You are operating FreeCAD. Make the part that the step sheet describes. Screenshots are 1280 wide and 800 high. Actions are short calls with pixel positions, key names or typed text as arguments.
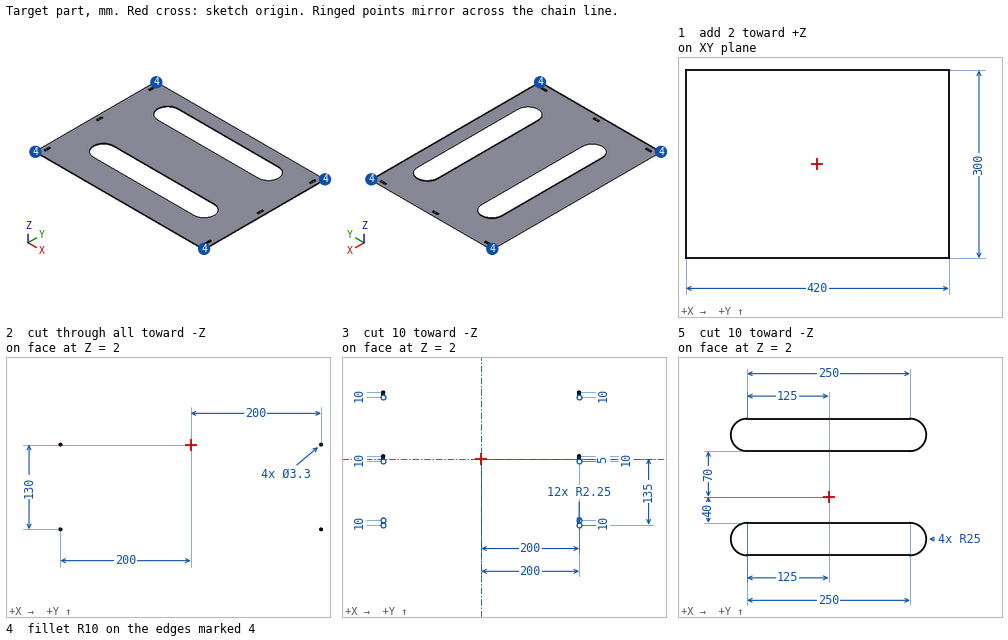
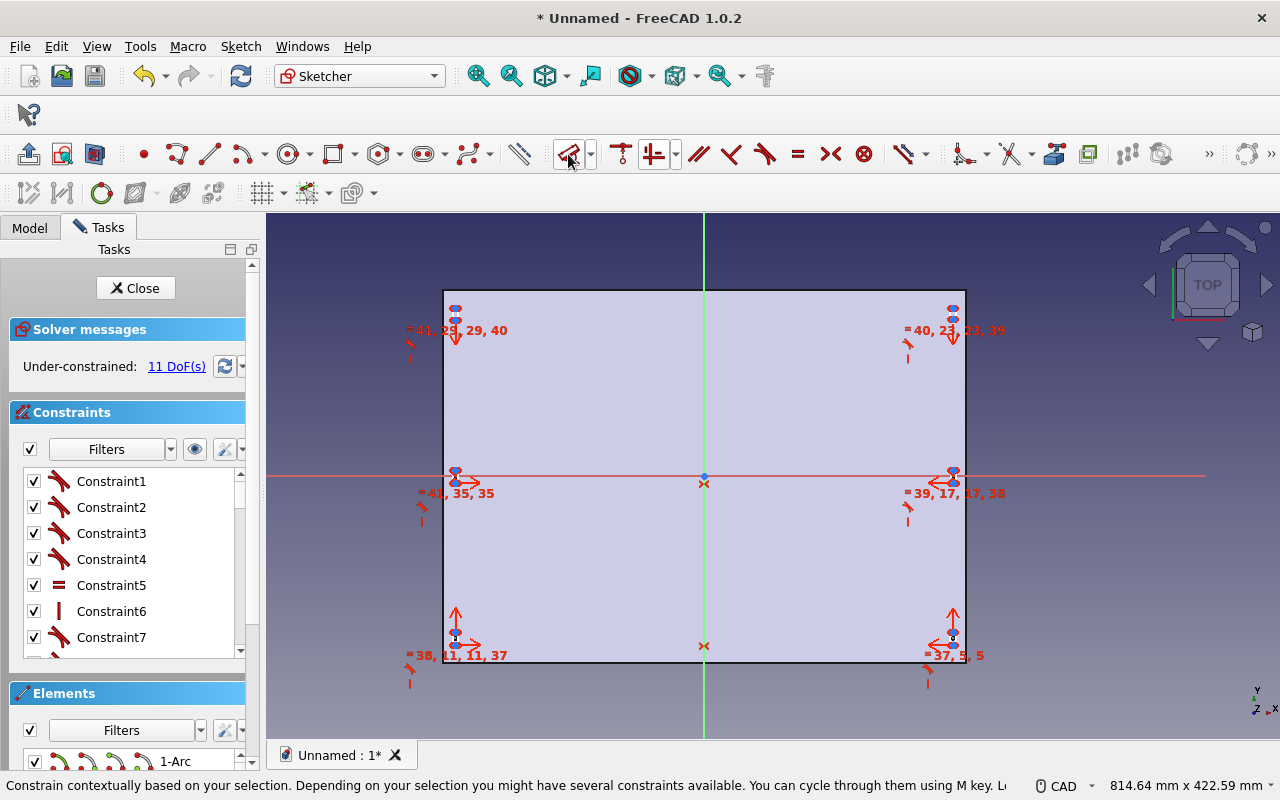
scroll(953, 648, up, 14)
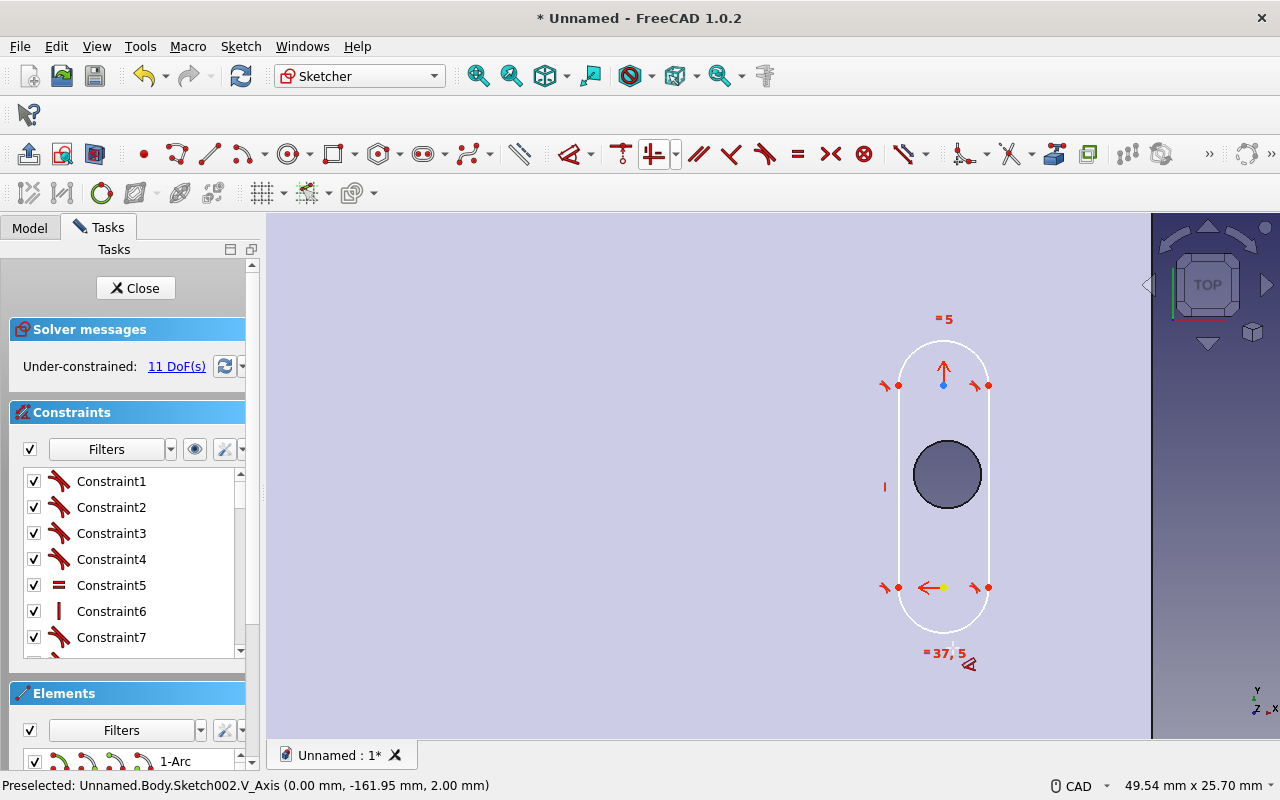
click(944, 633)
click(944, 665)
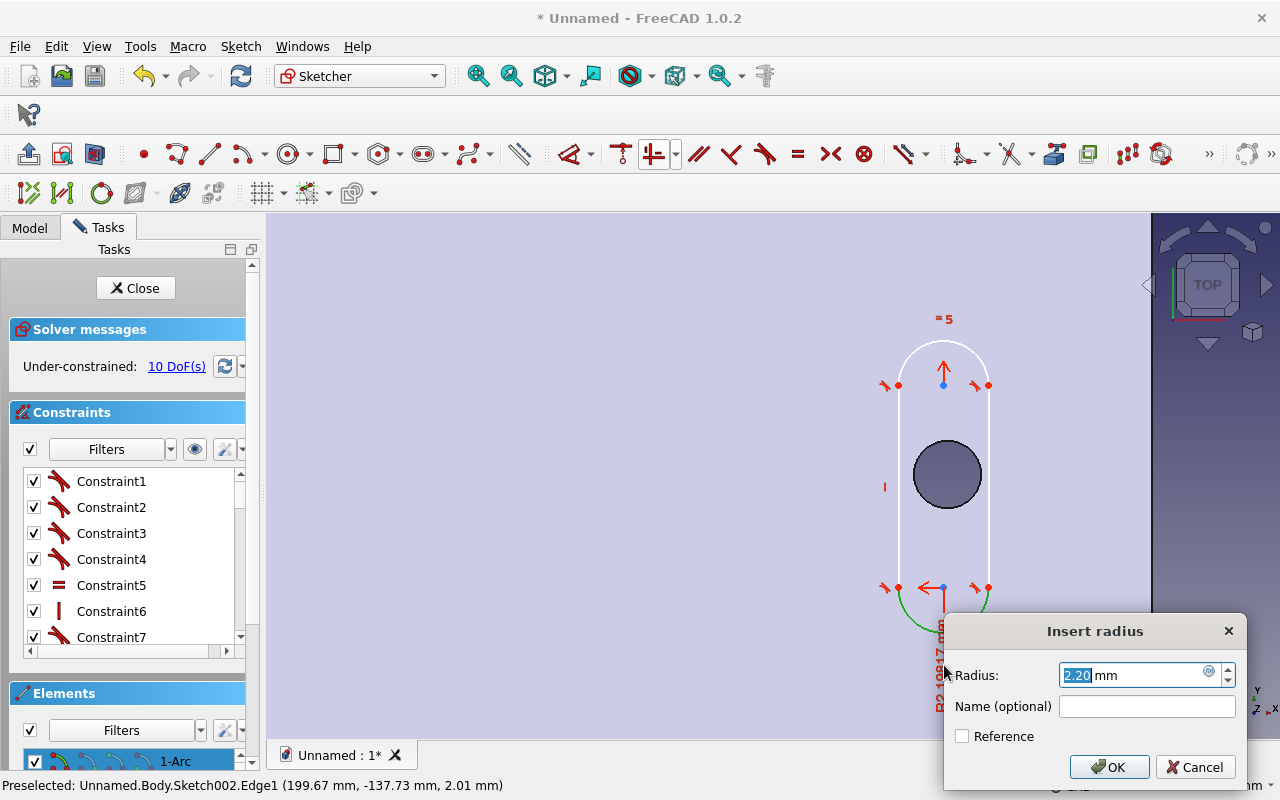
text(2.25)
key(Return)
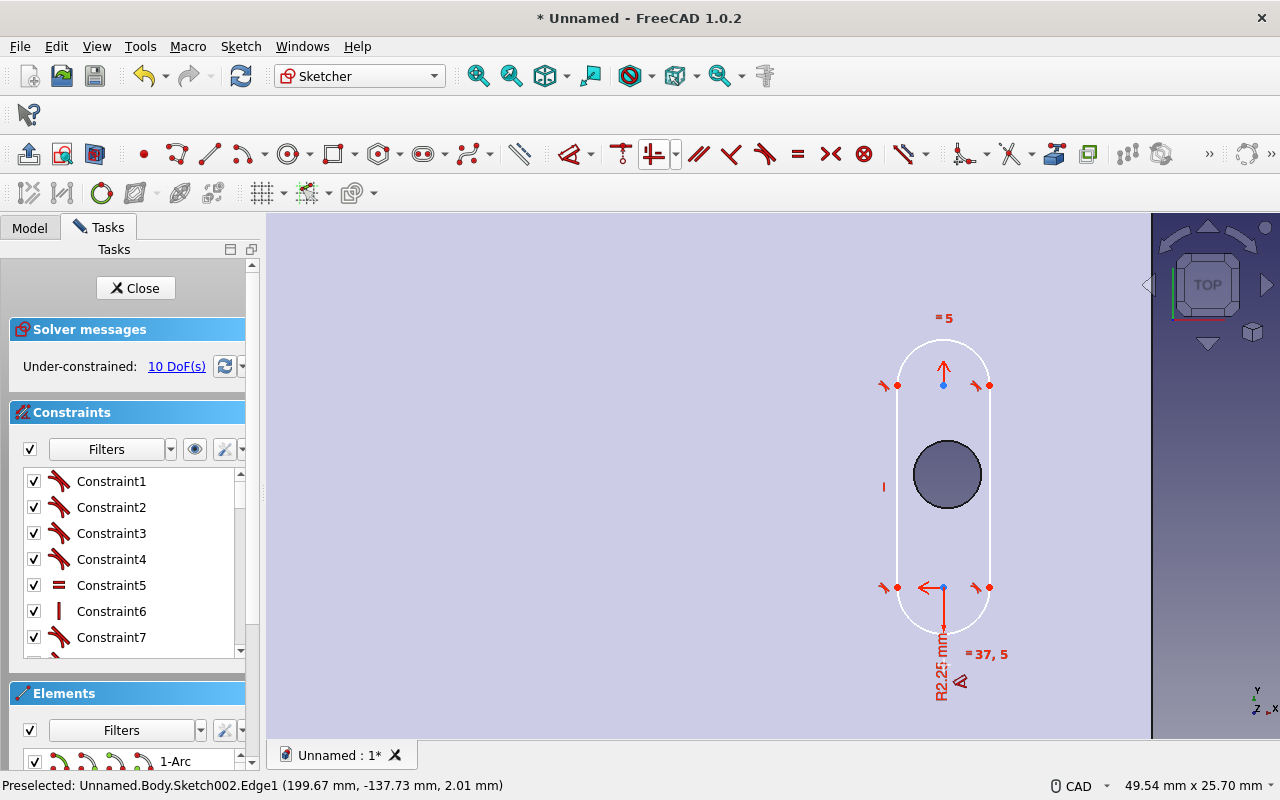
scroll(954, 648, down, 14)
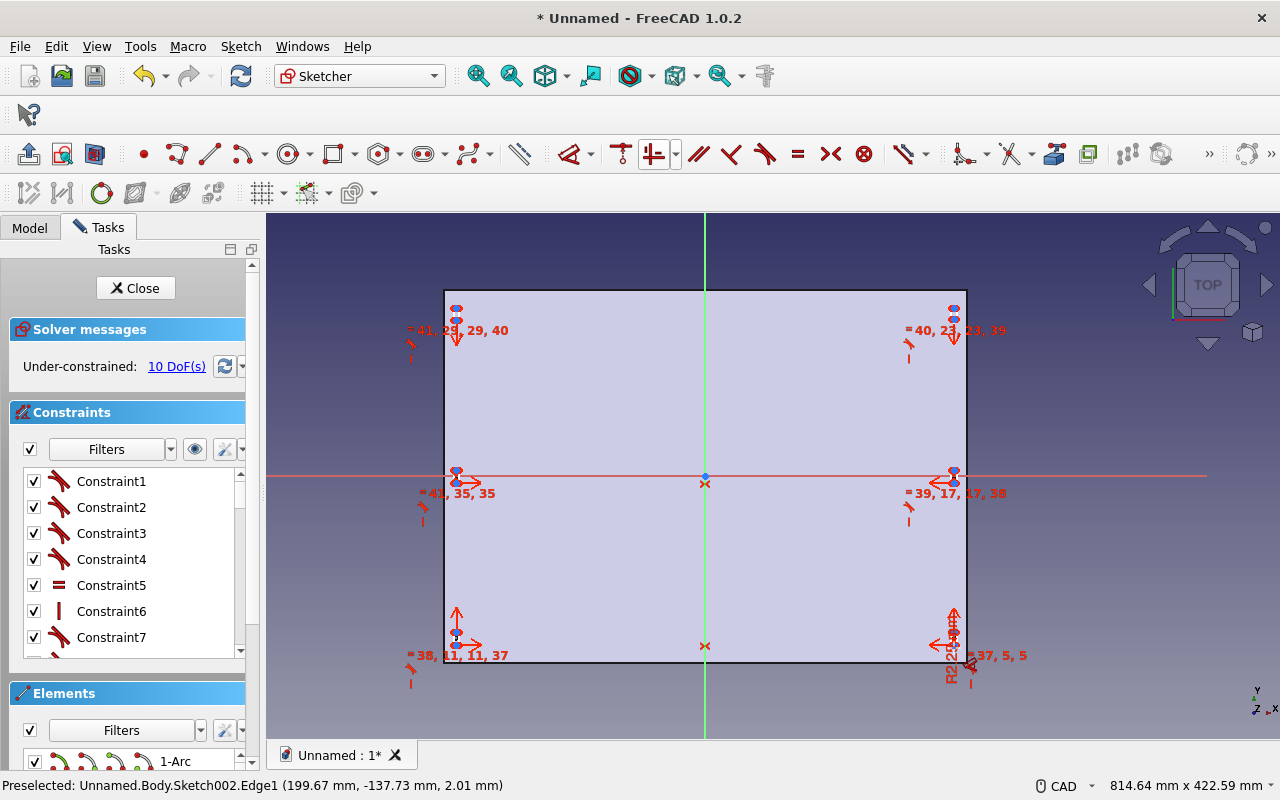
scroll(951, 641, up, 7)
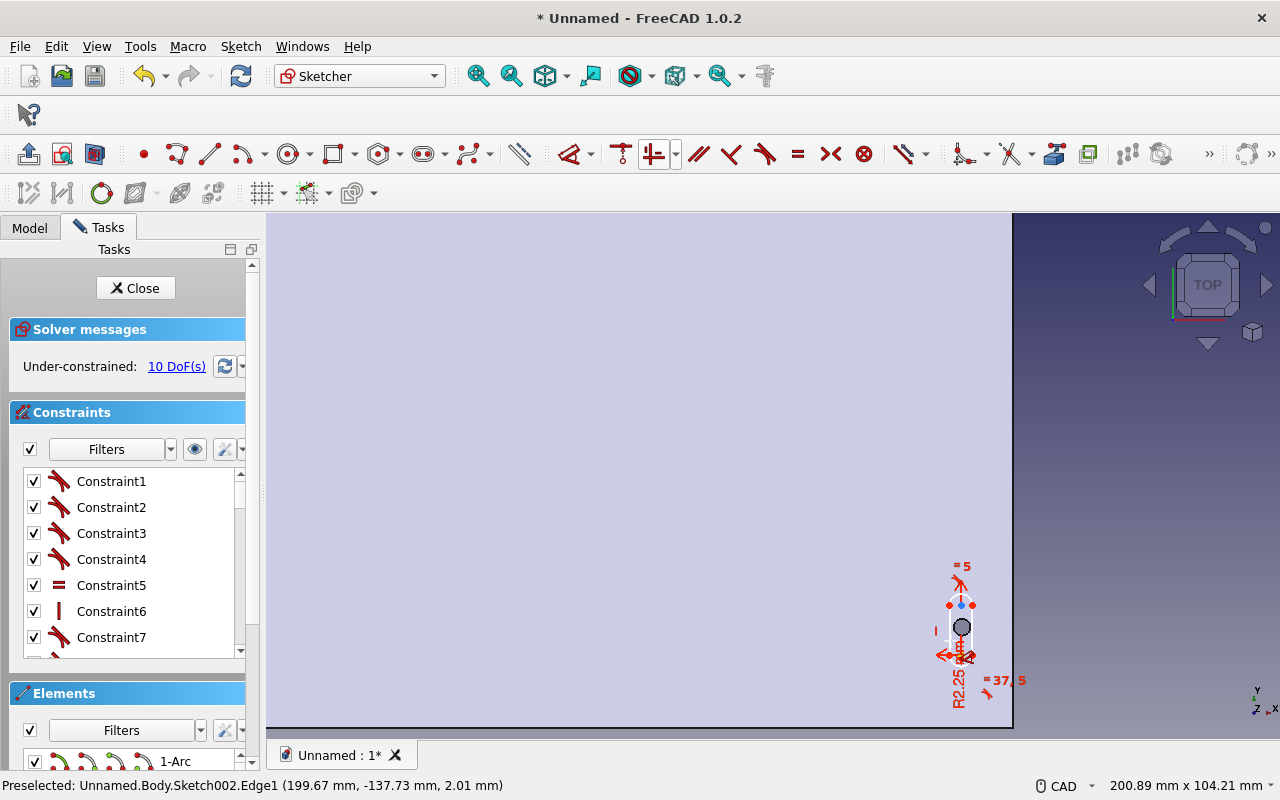
click(950, 640)
click(916, 630)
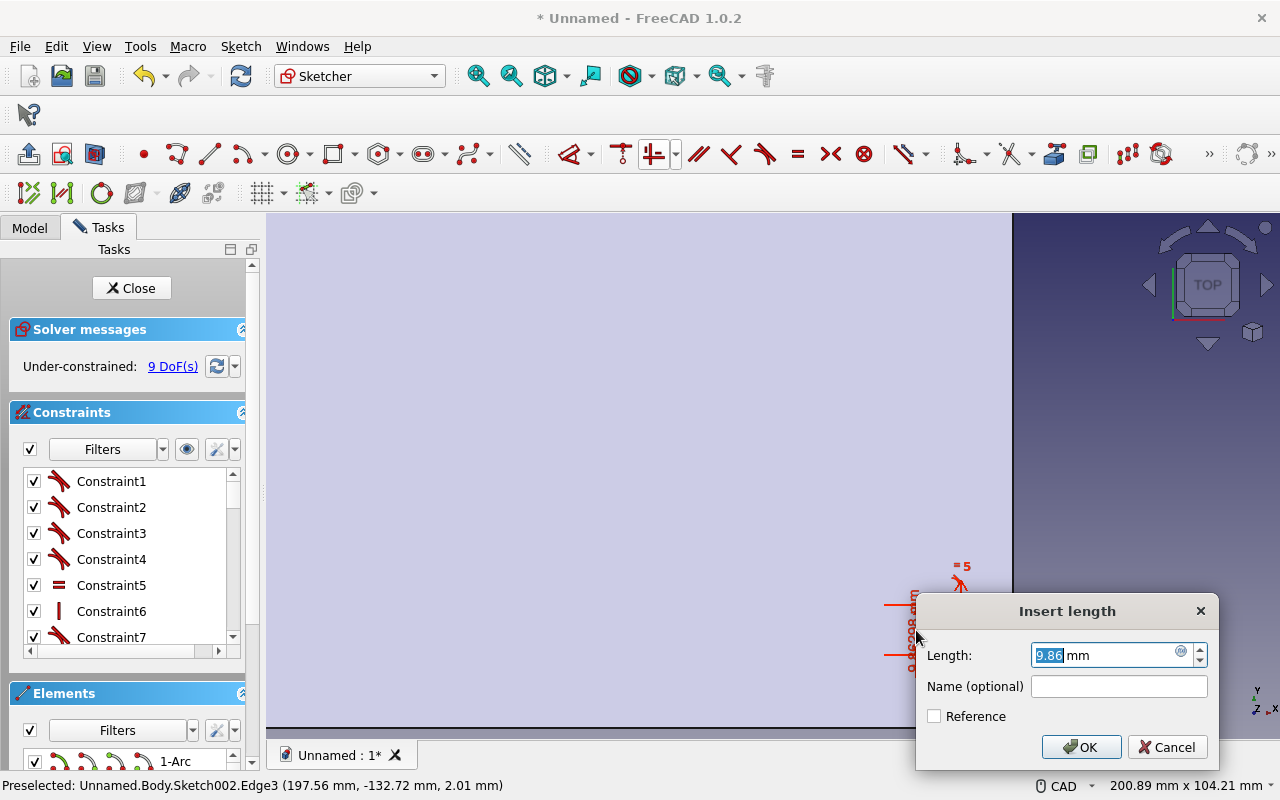
text(10)
key(Return)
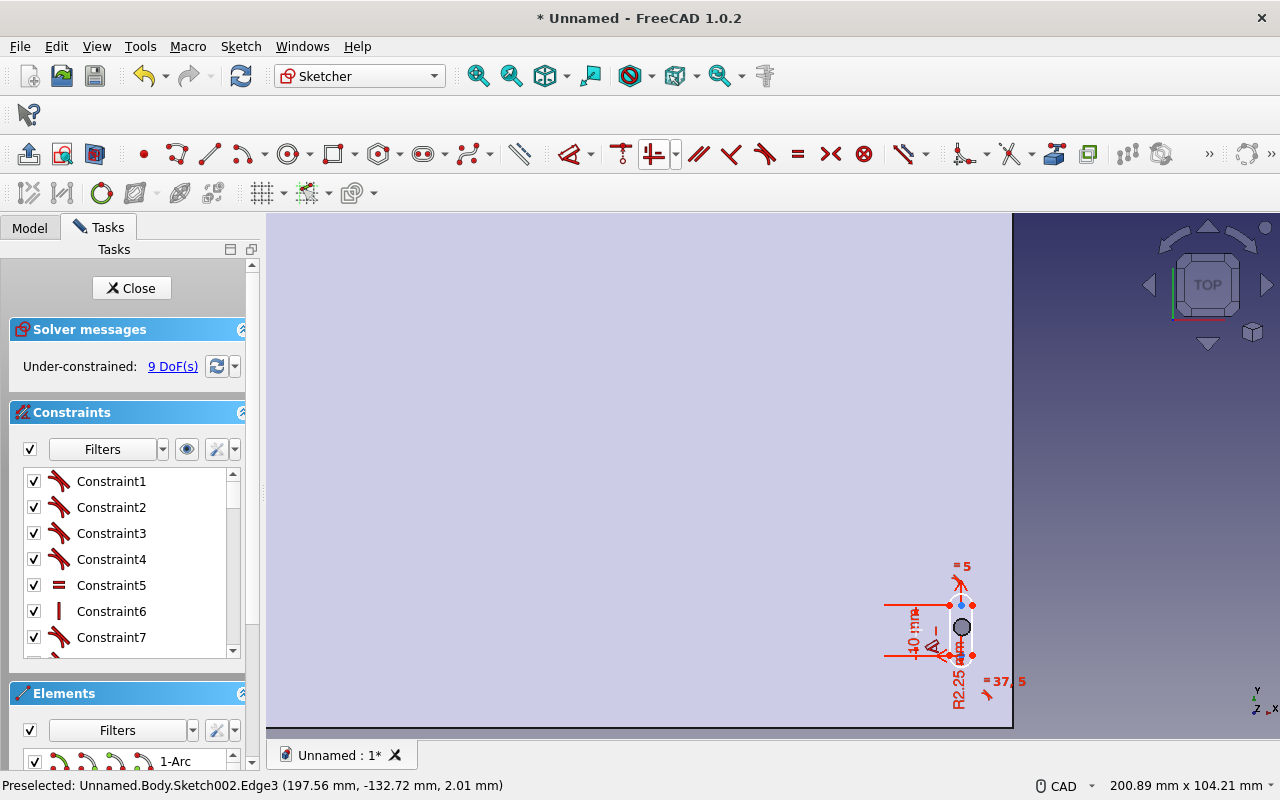
scroll(951, 641, down, 7)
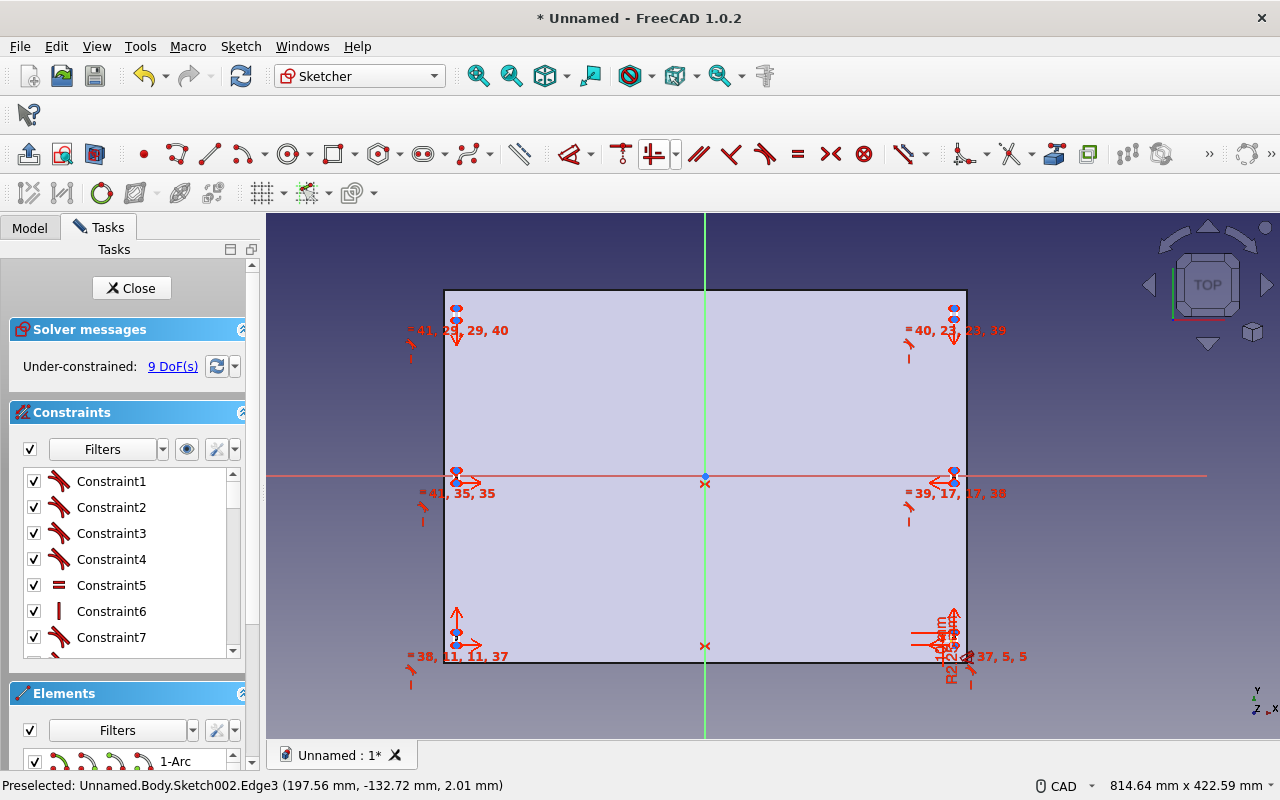
scroll(454, 642, up, 7)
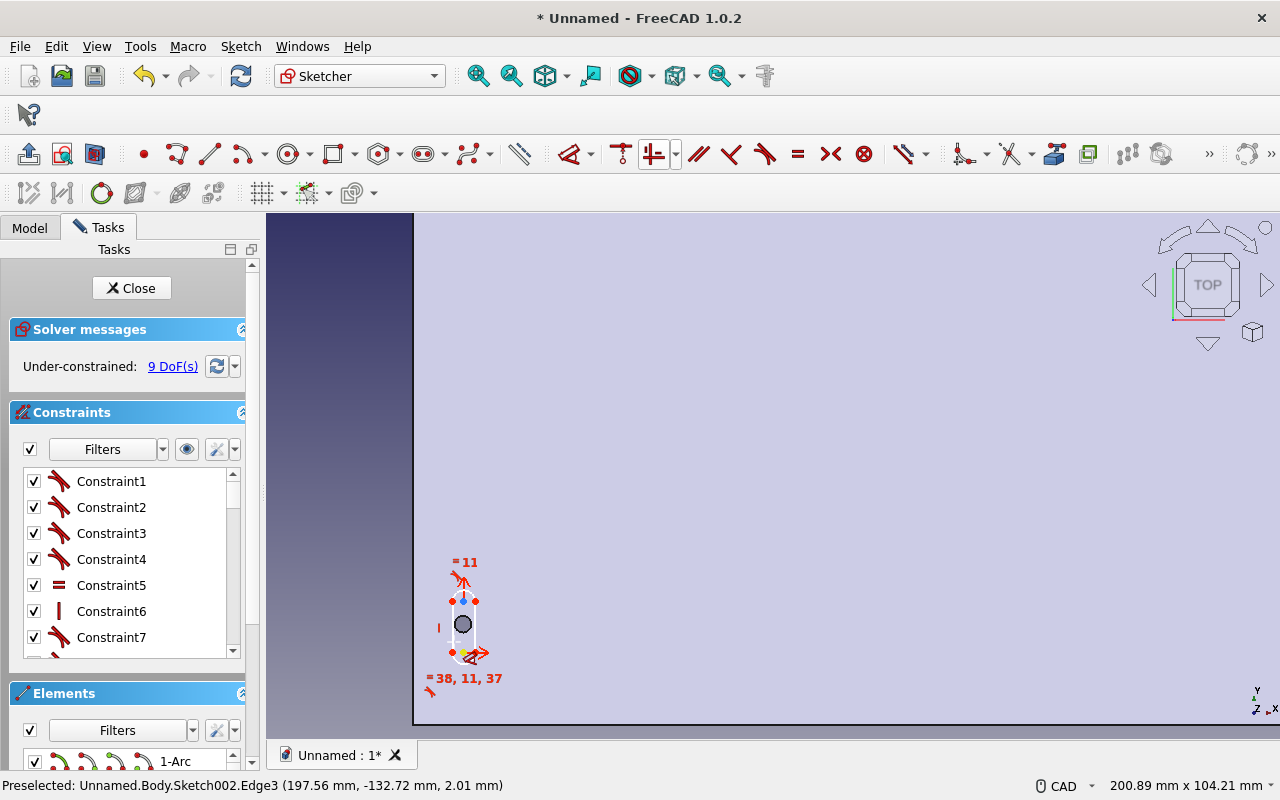
click(453, 638)
click(419, 627)